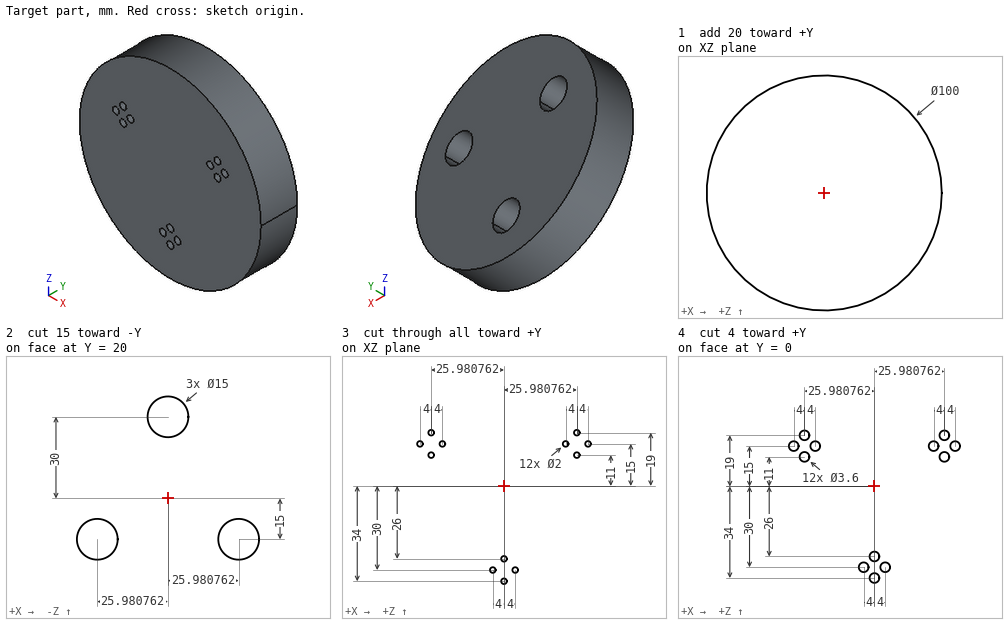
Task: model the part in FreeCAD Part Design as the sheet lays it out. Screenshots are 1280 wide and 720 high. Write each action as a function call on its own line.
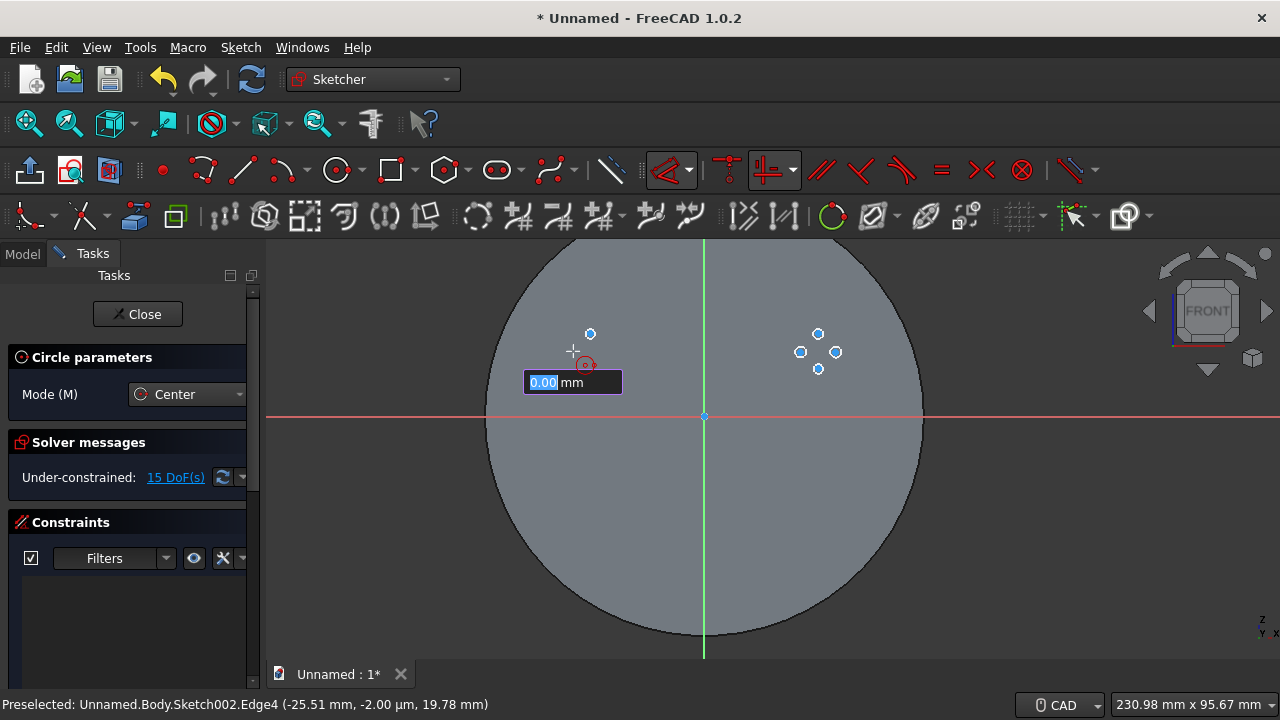
scroll(576, 348, up, 7)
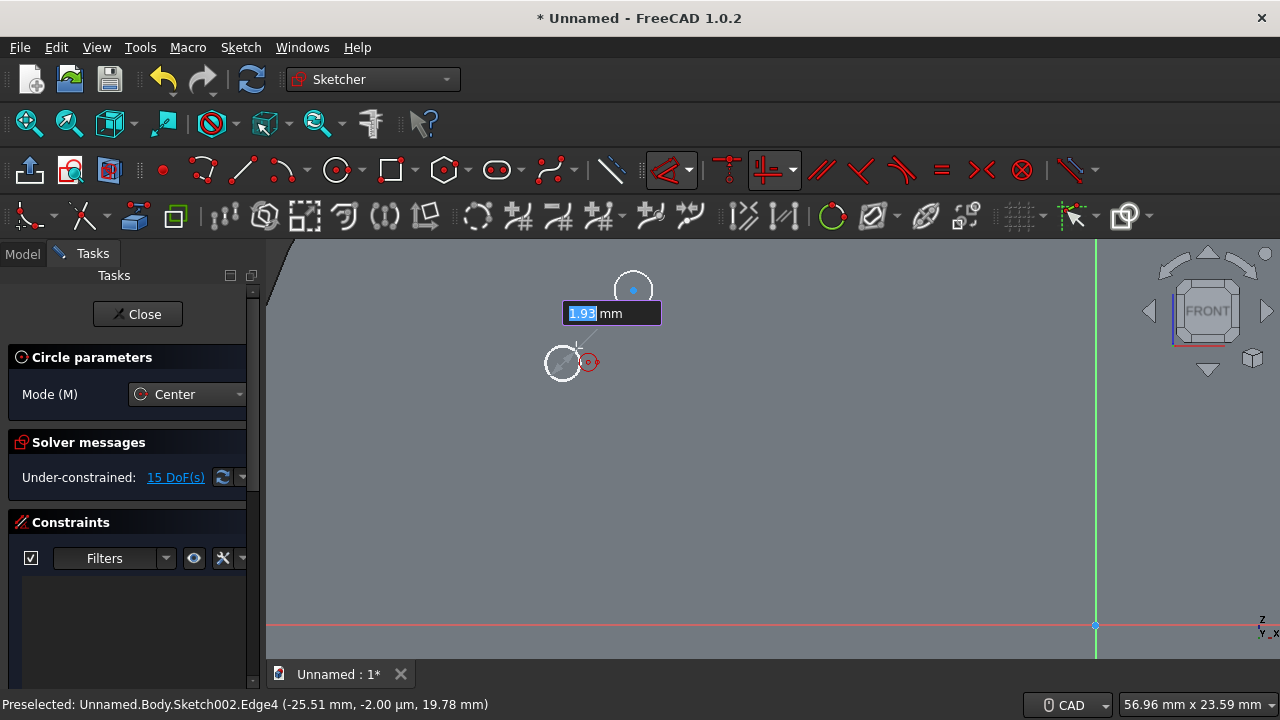
click(575, 345)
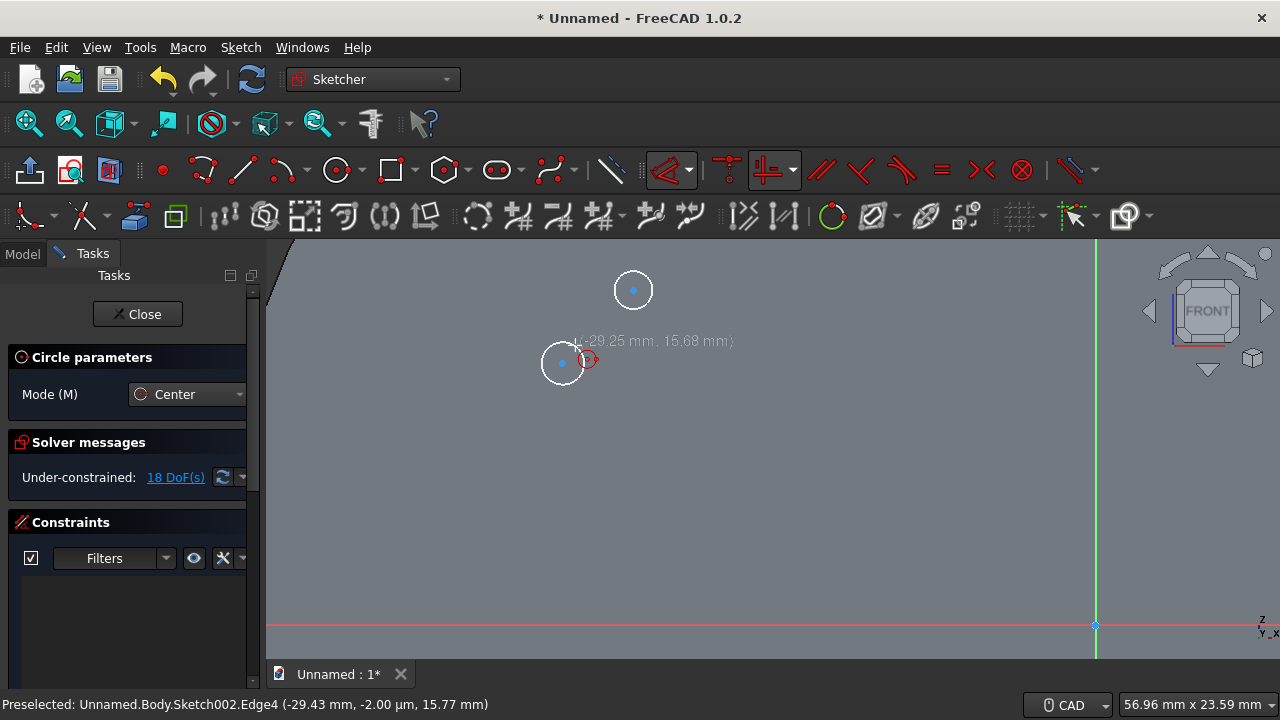
scroll(633, 429, up, 2)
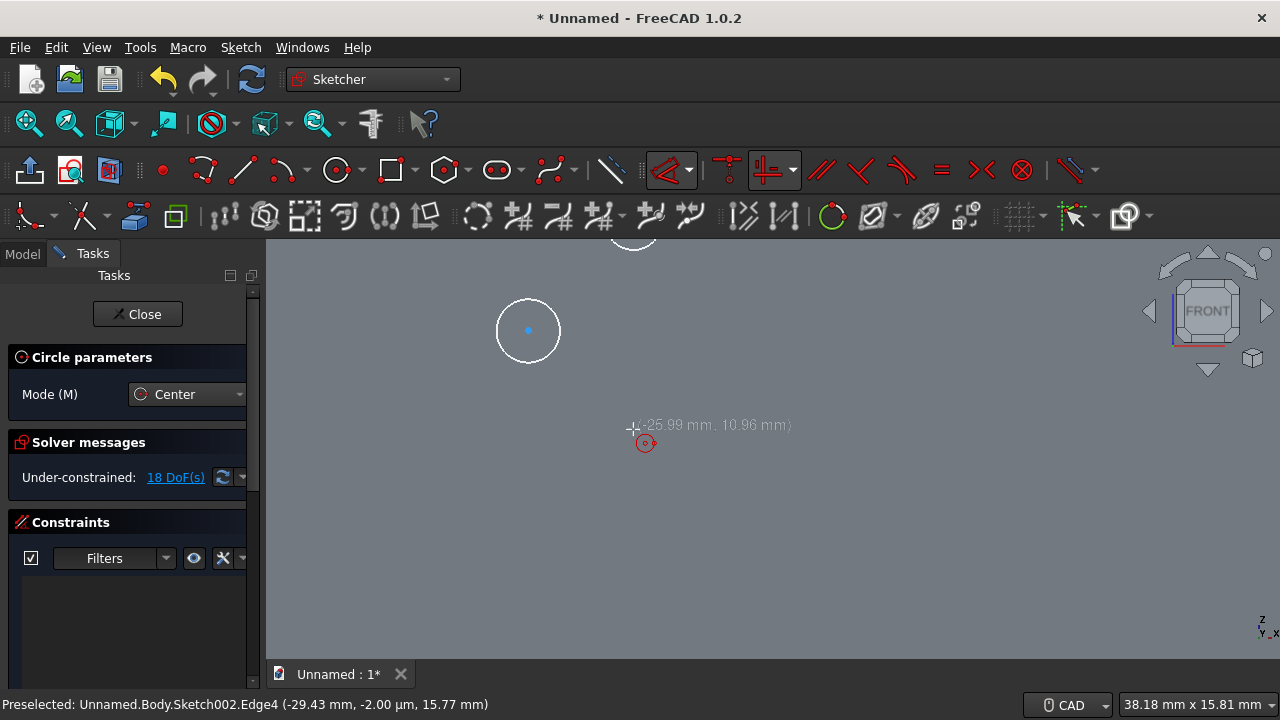
scroll(582, 356, down, 9)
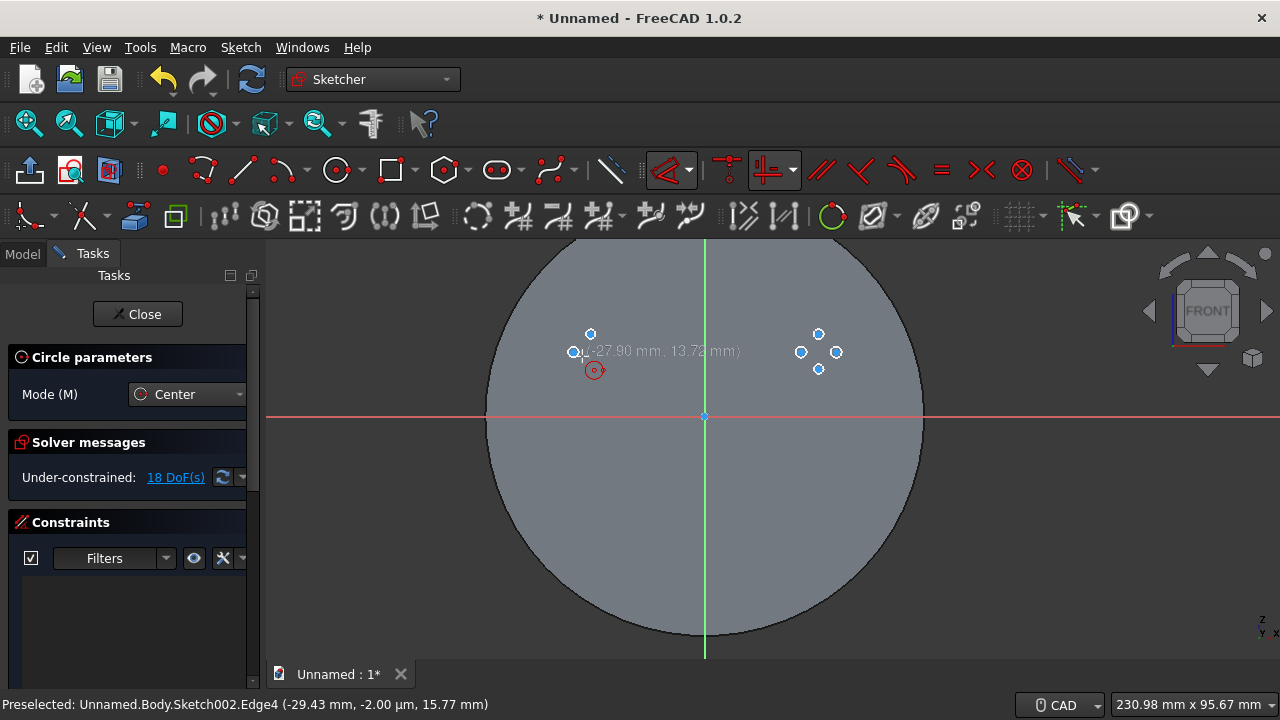
click(591, 368)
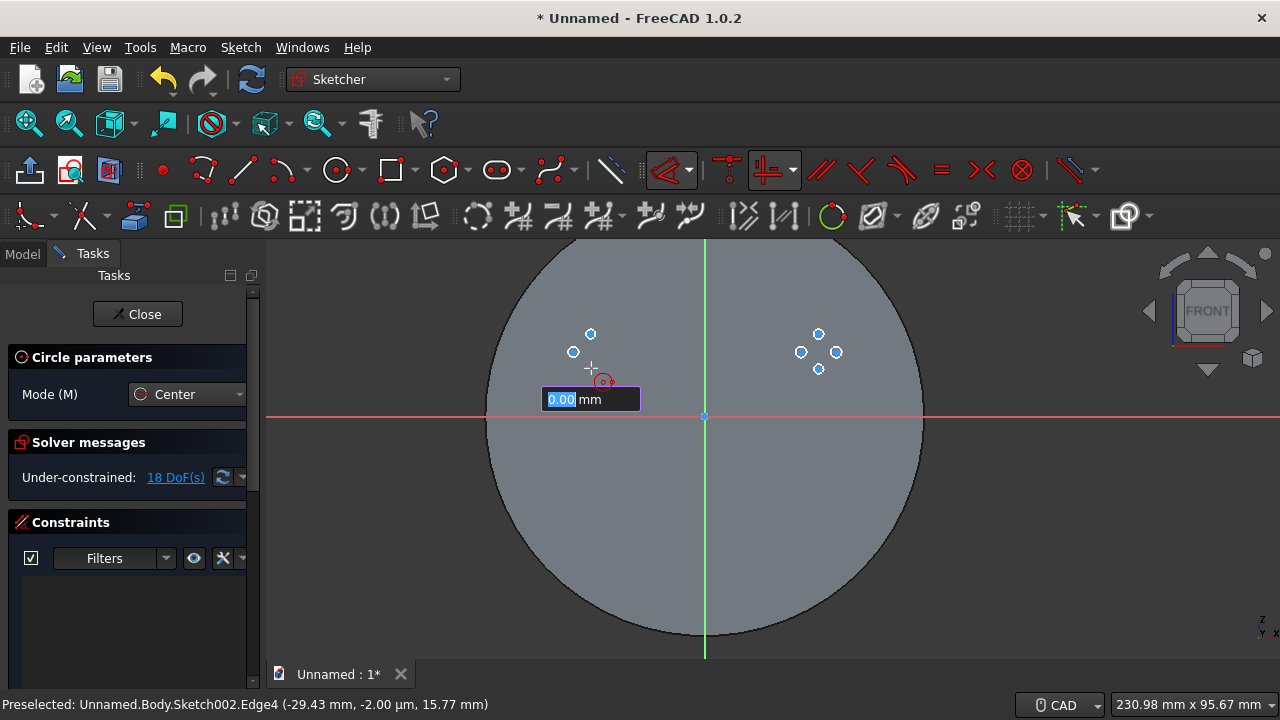
scroll(594, 365, up, 7)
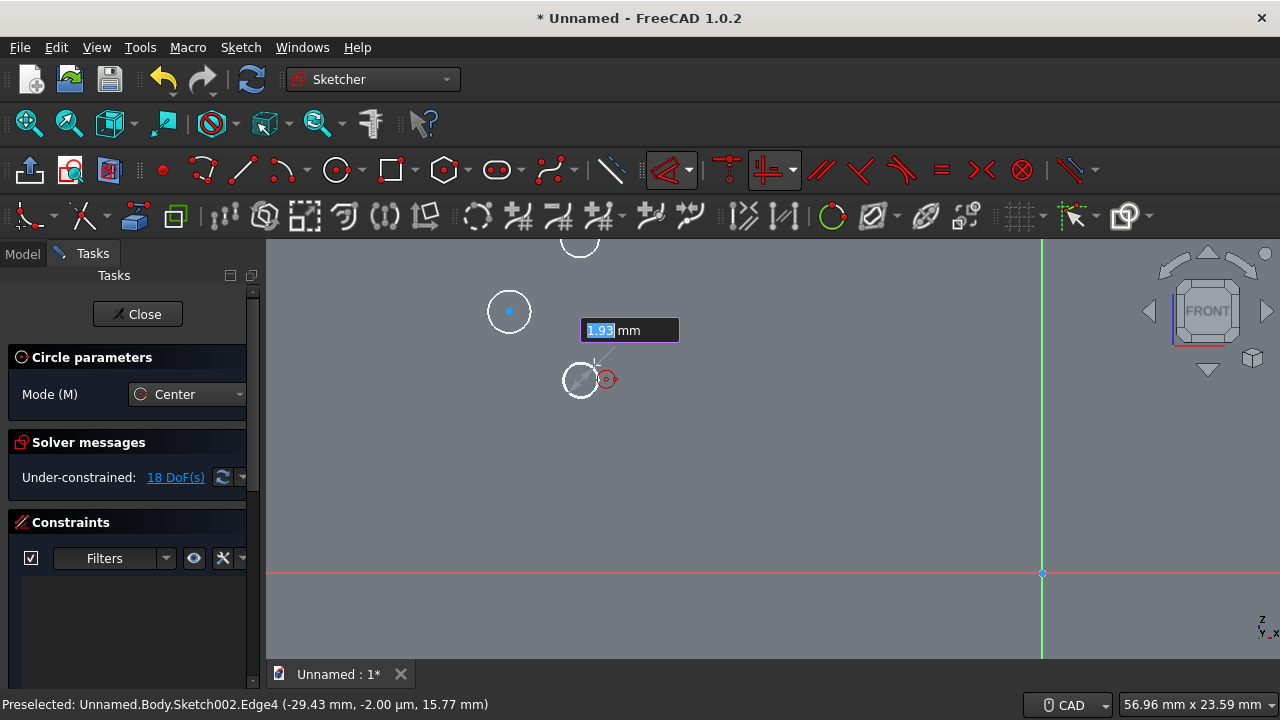
click(592, 365)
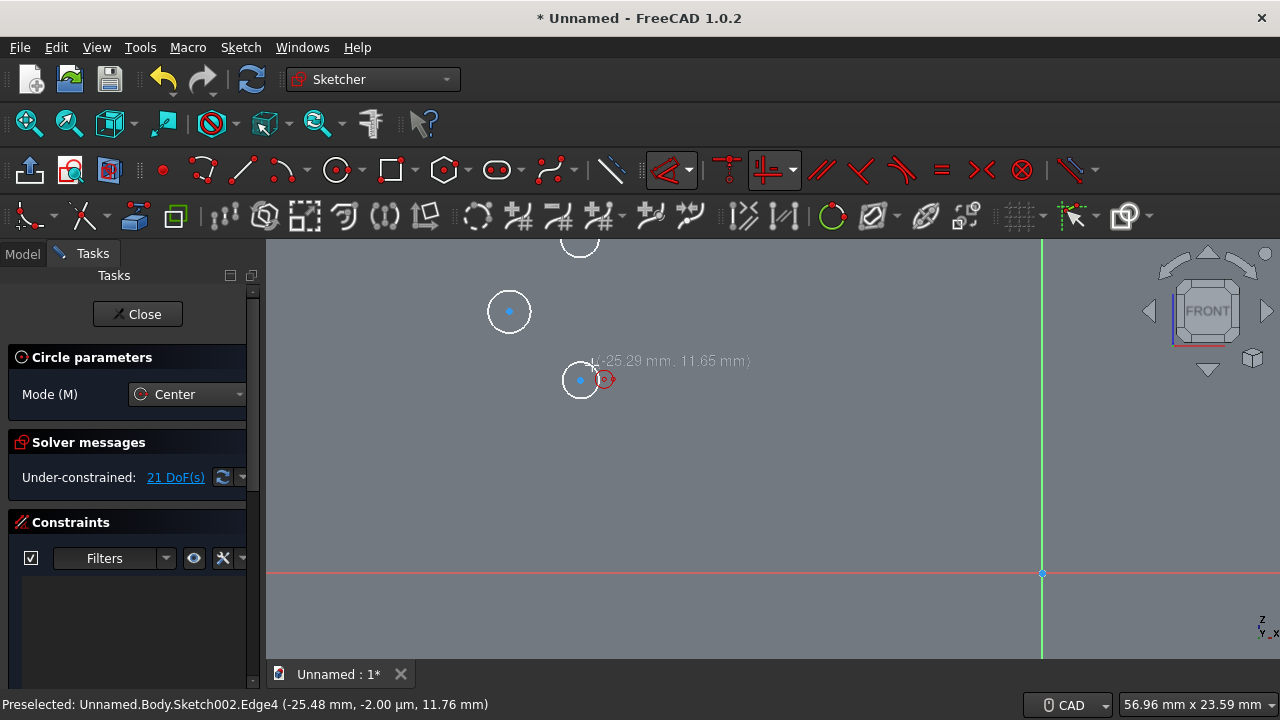
scroll(651, 306, up, 2)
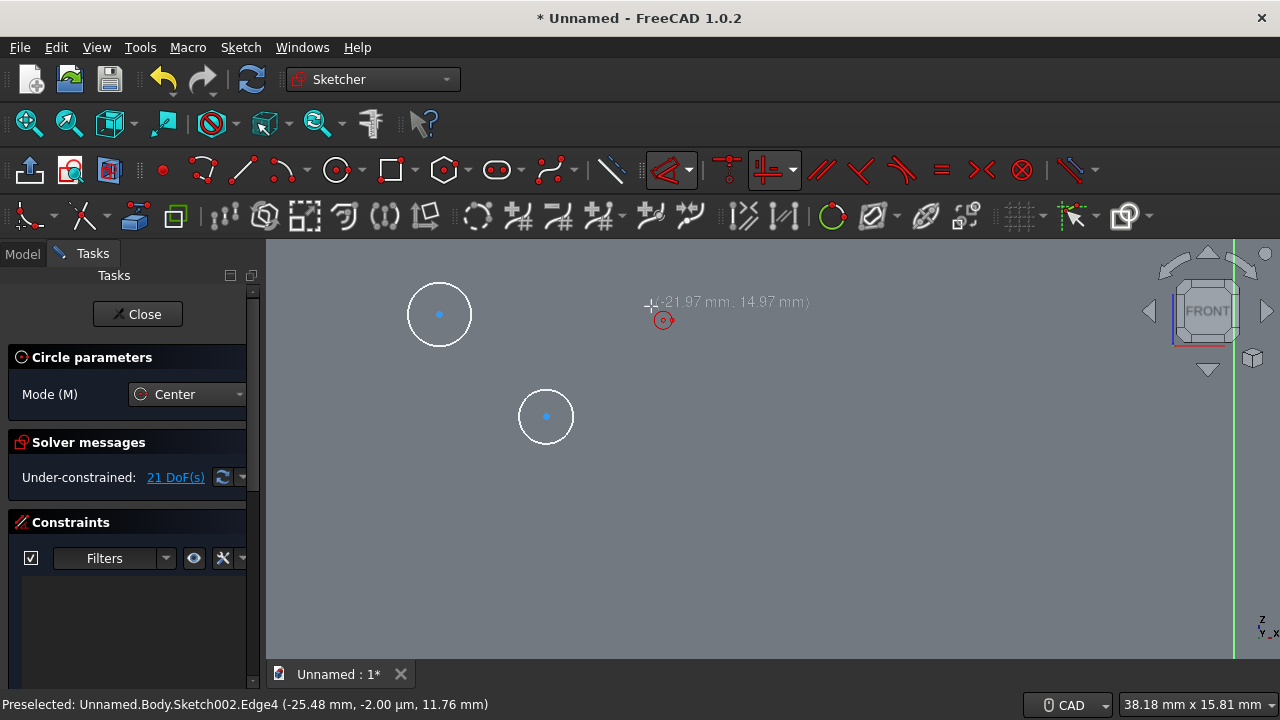
scroll(600, 359, down, 9)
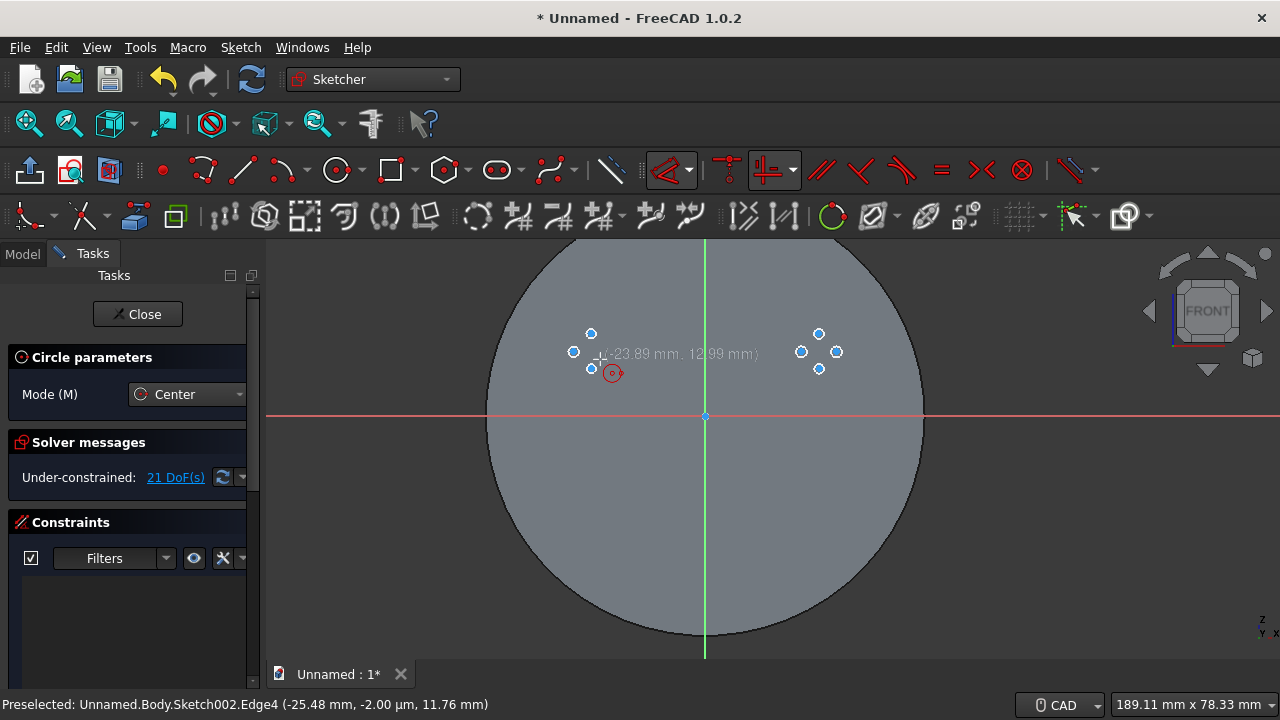
click(609, 351)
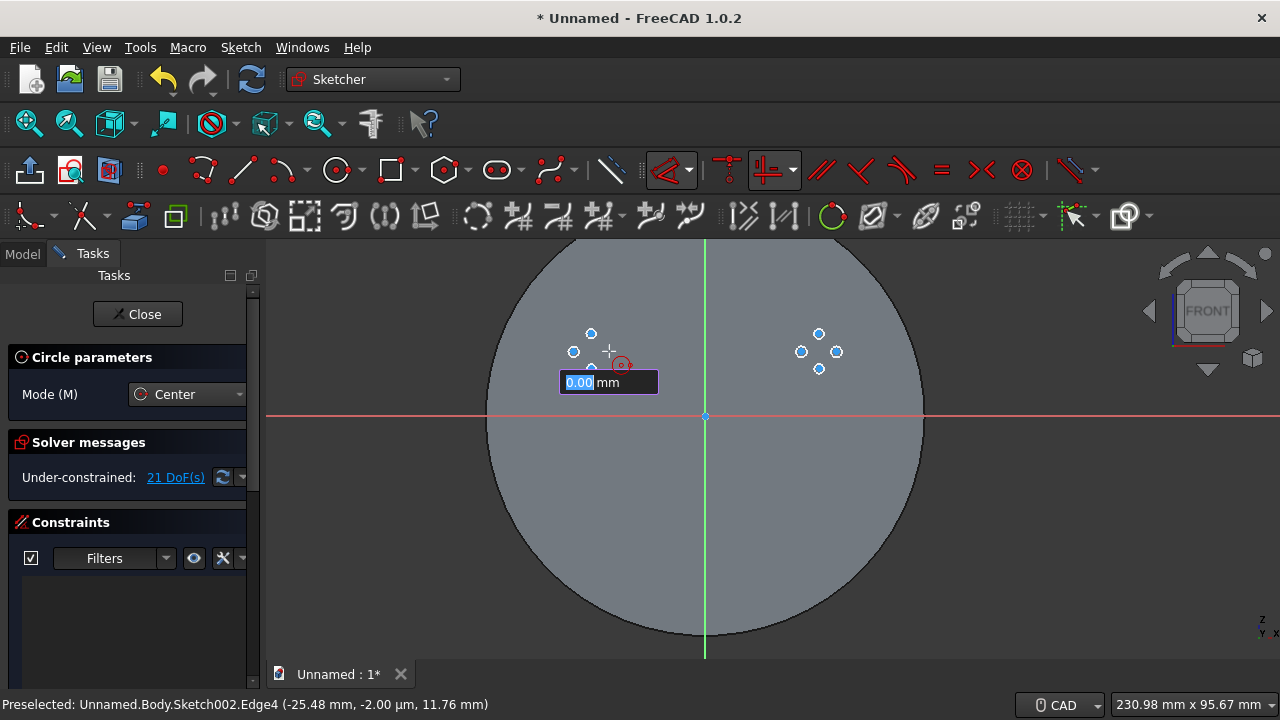
scroll(612, 347, up, 7)